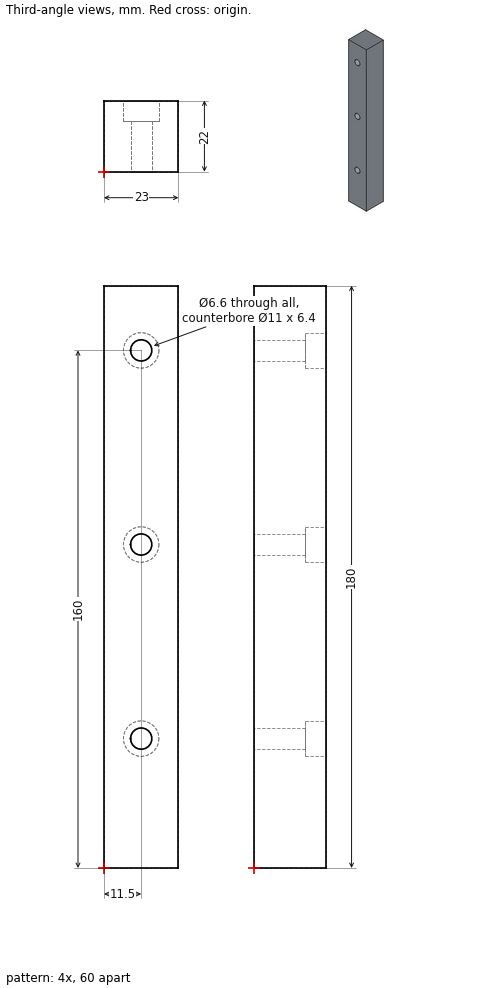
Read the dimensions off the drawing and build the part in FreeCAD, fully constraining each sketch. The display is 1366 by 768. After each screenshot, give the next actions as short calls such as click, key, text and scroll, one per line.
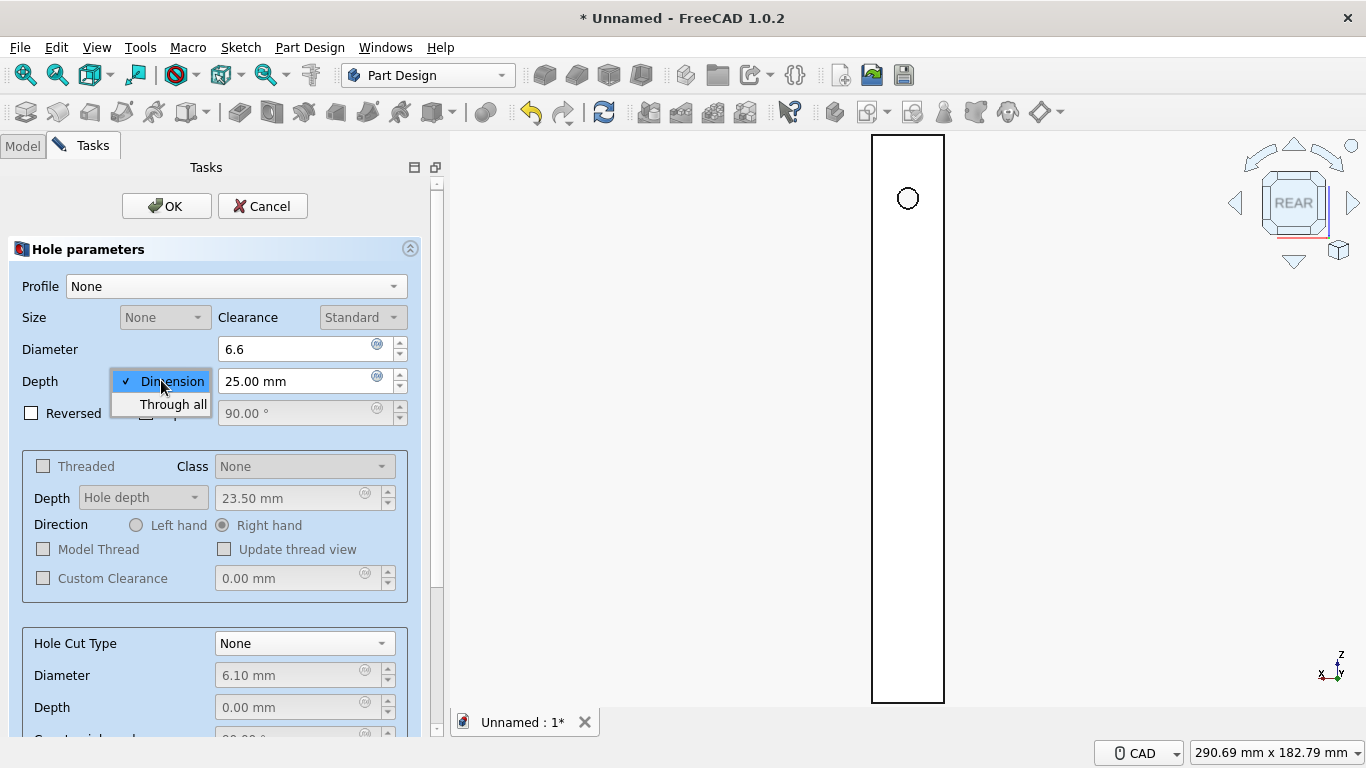
click(160, 404)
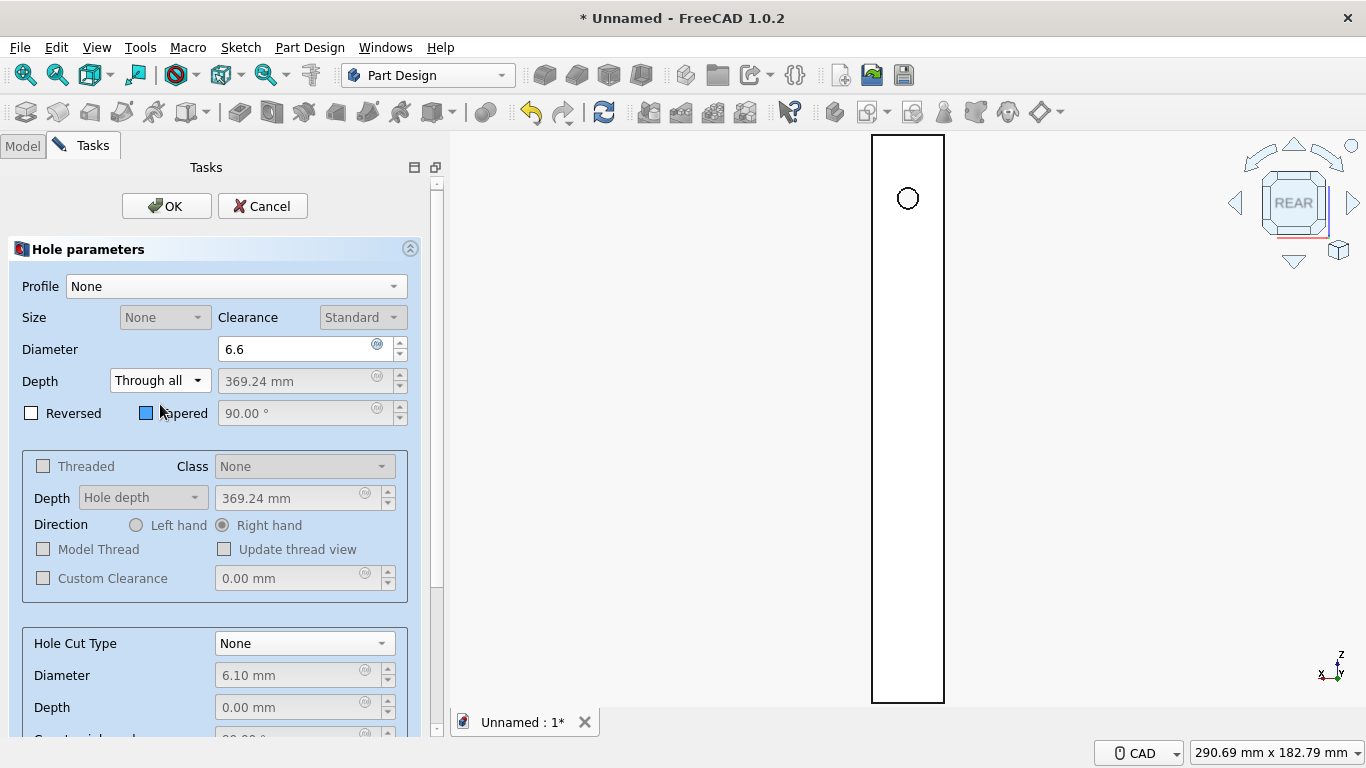
click(306, 644)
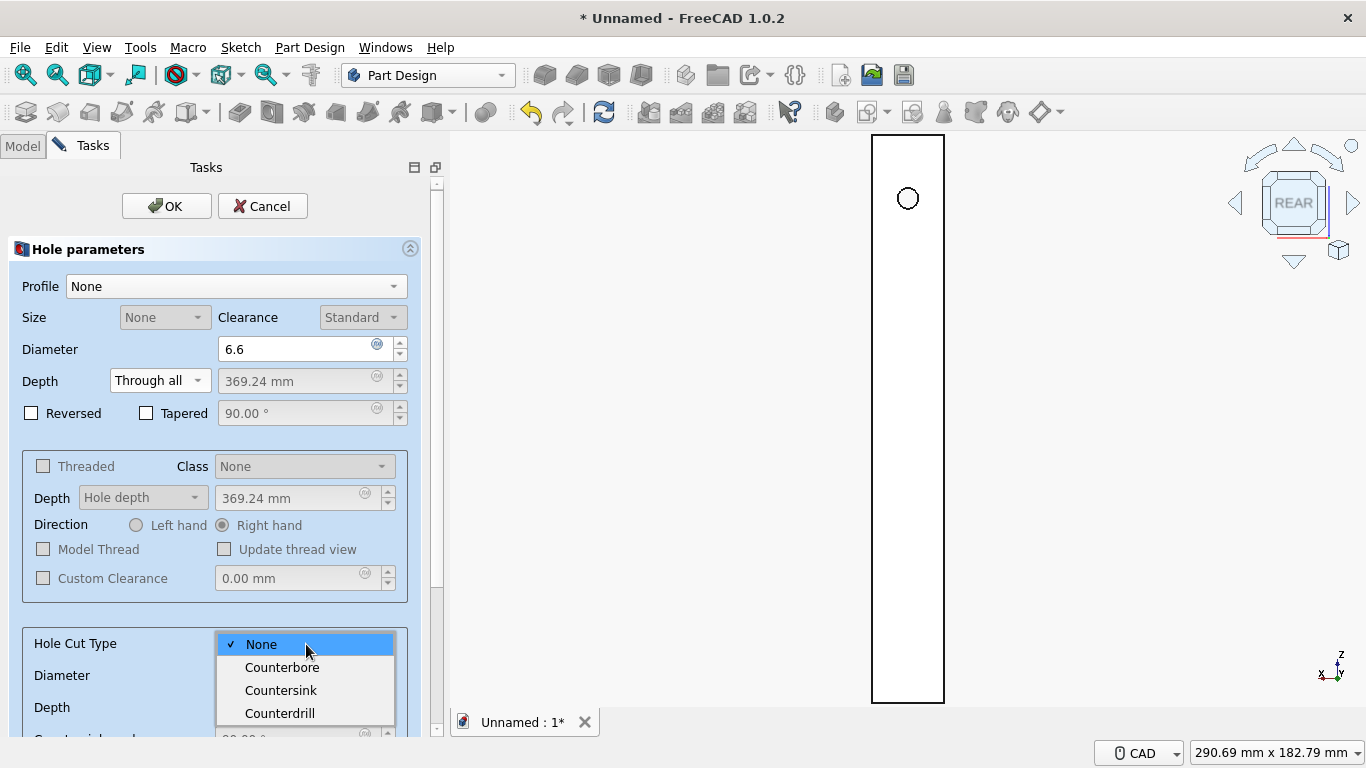
click(304, 668)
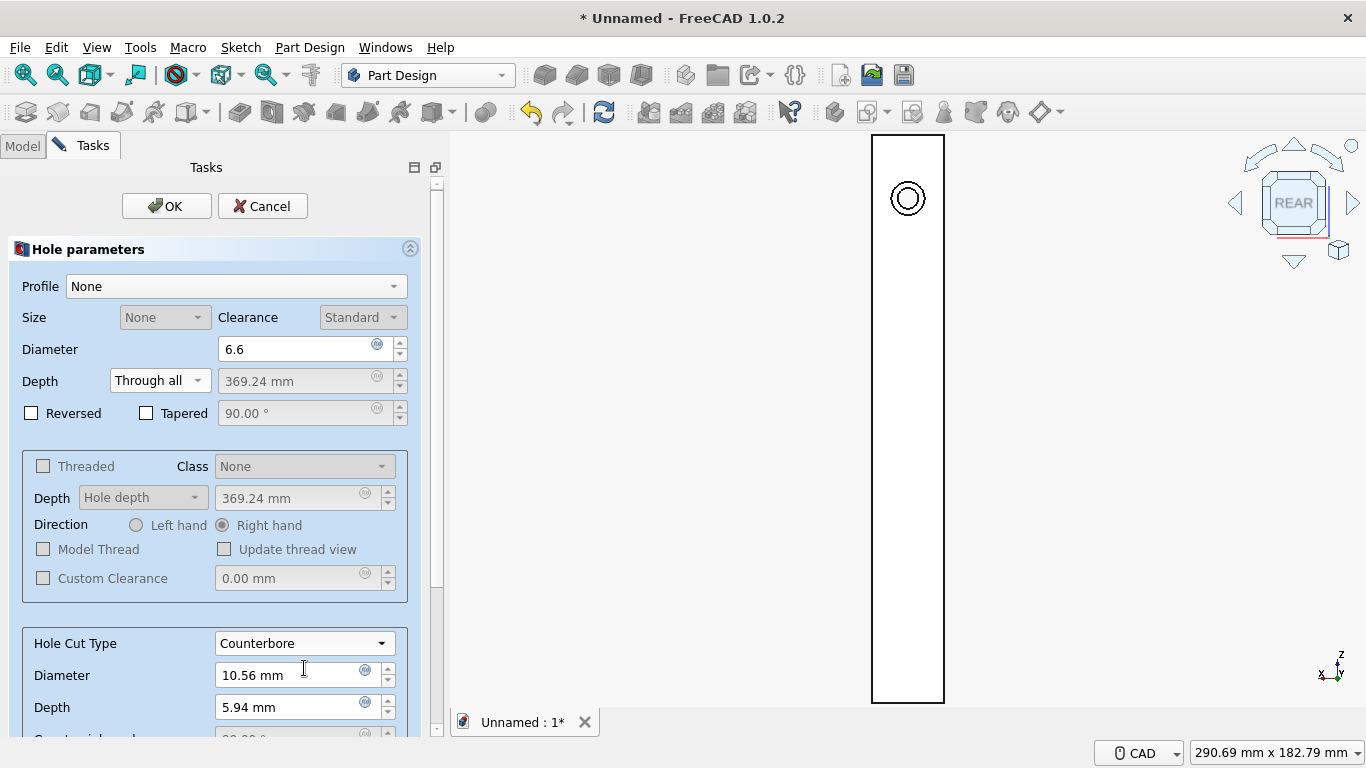
triple_click(298, 675)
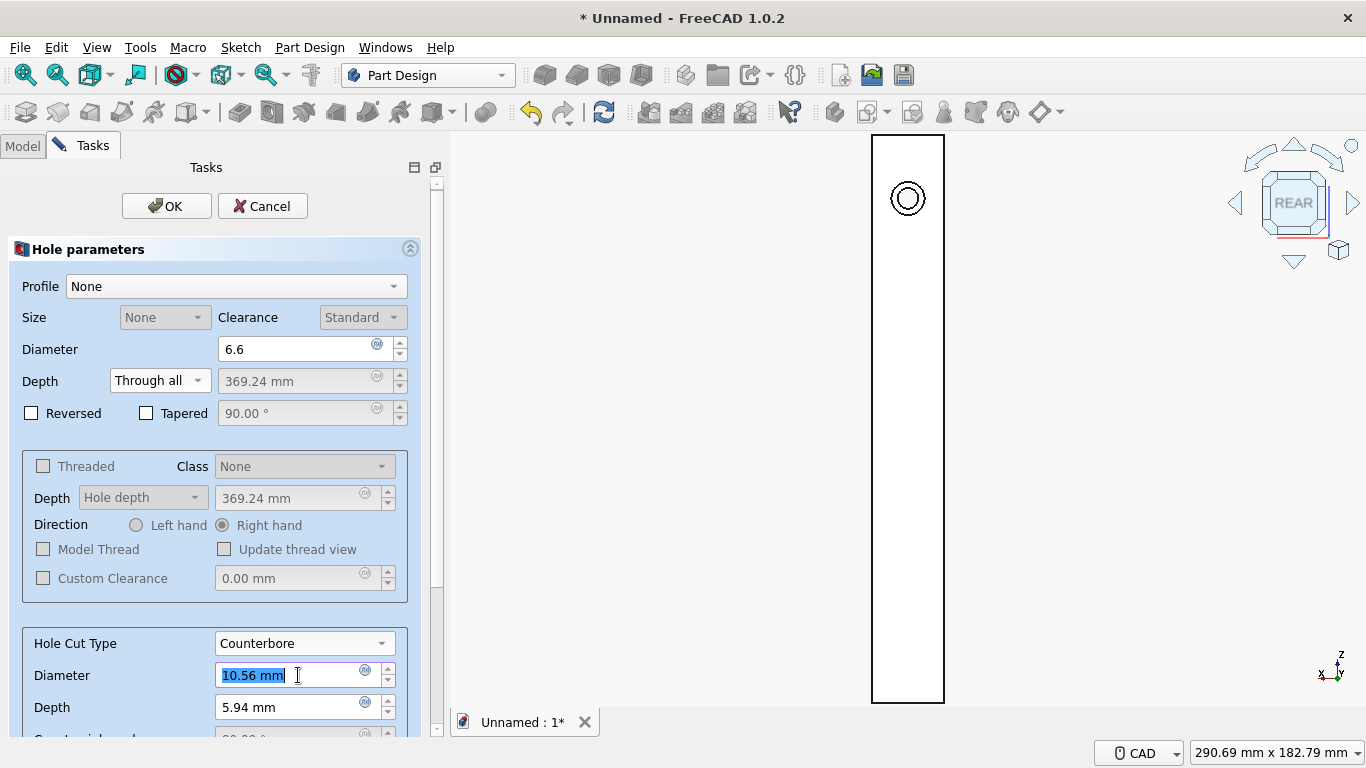
text(11)
key(Tab)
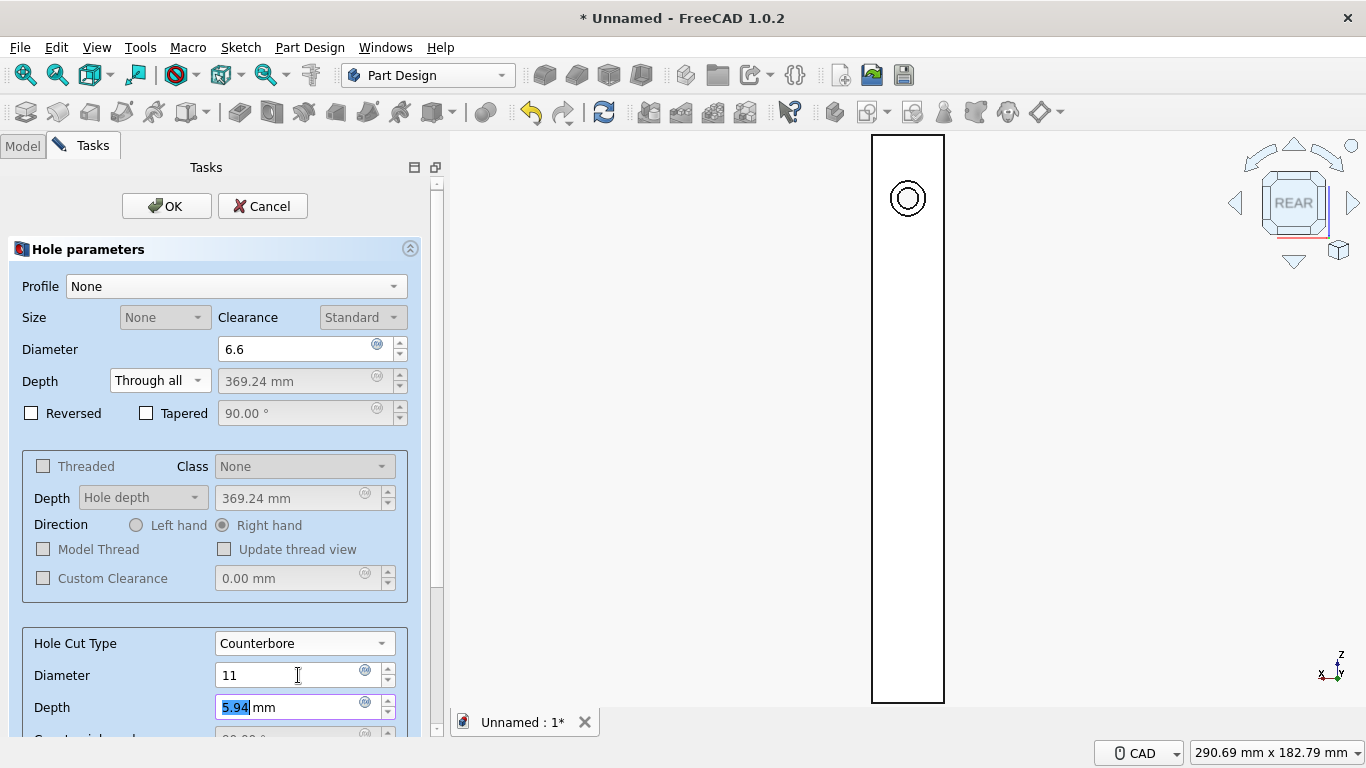
text(6.4)
key(Tab)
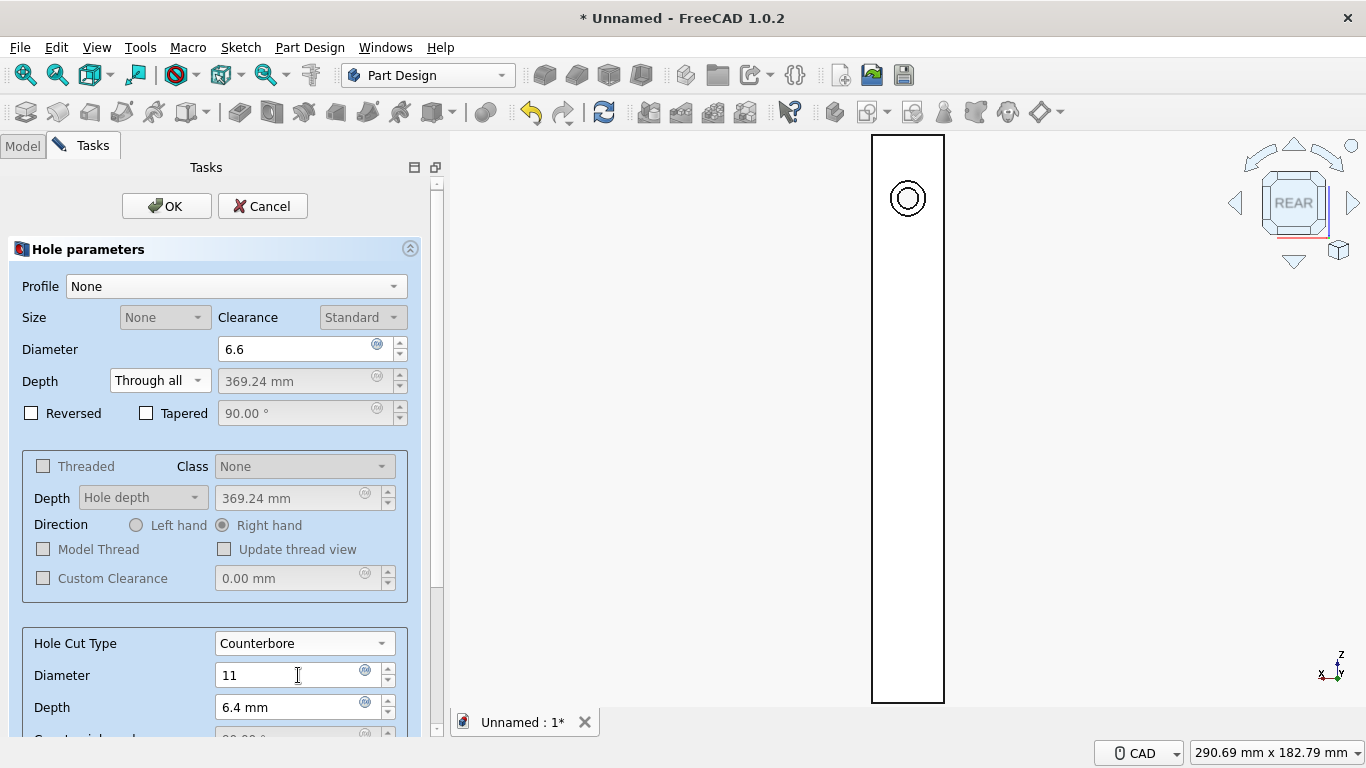
click(167, 206)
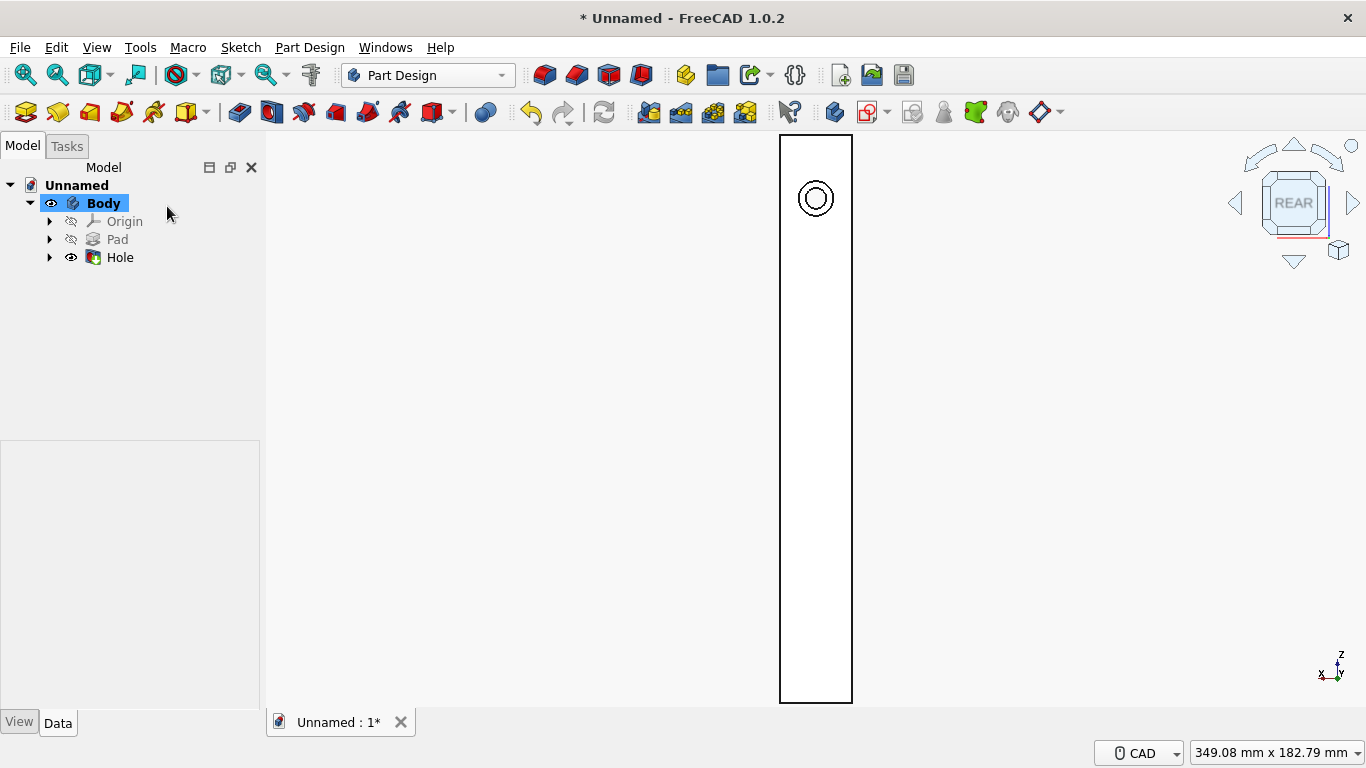
click(116, 257)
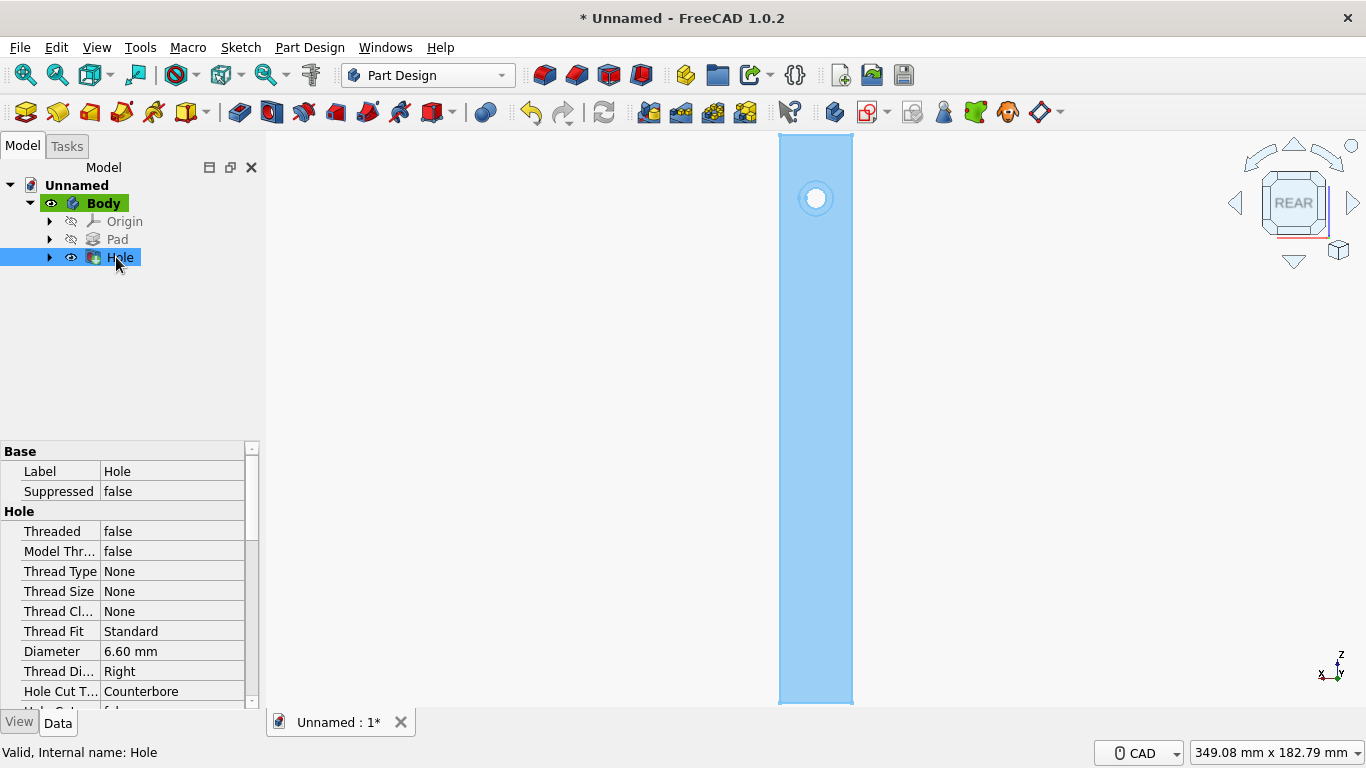
click(682, 112)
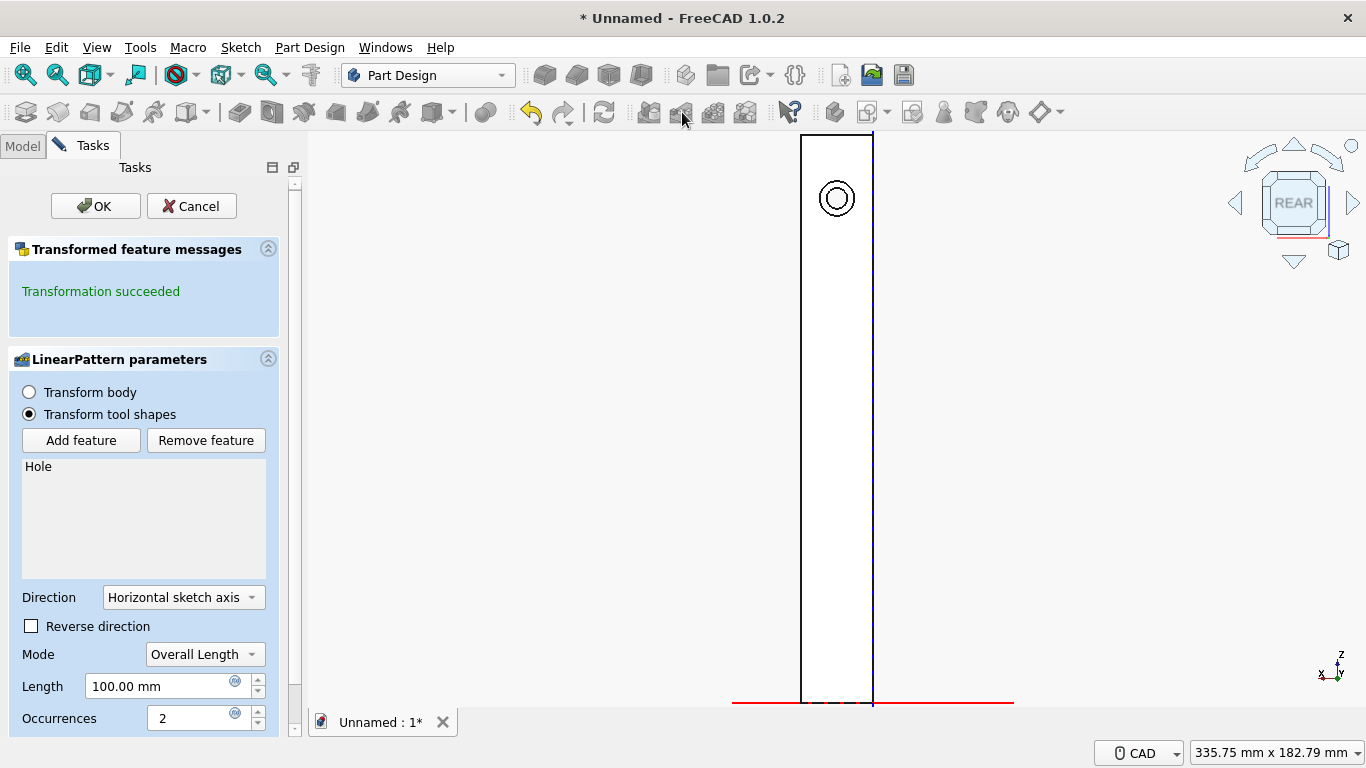
click(184, 598)